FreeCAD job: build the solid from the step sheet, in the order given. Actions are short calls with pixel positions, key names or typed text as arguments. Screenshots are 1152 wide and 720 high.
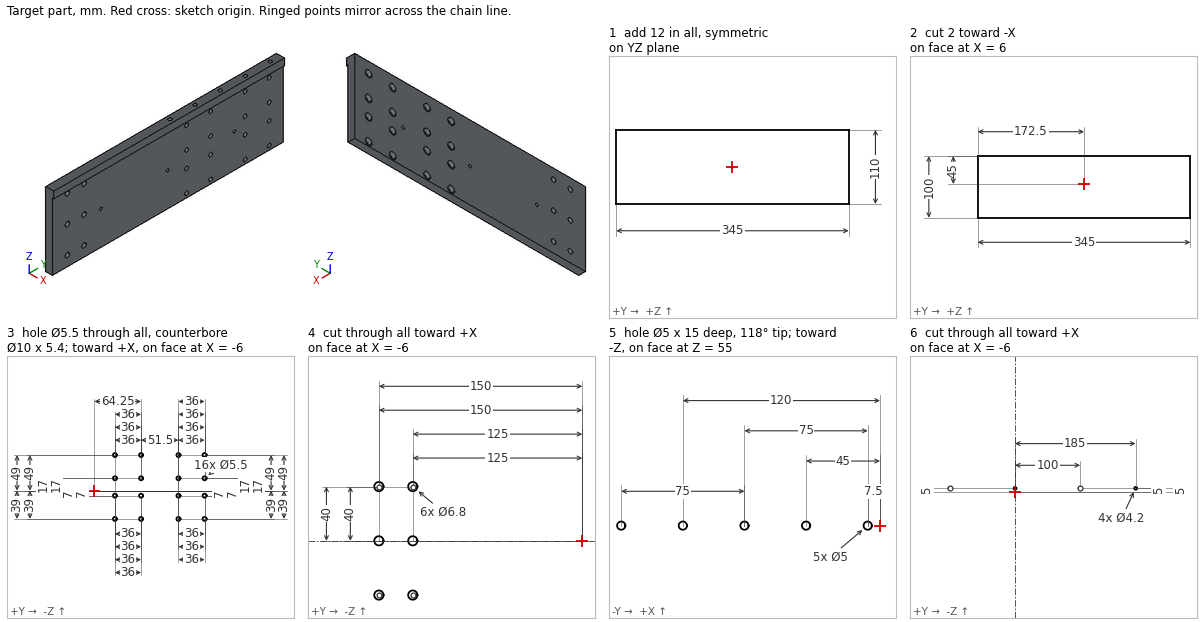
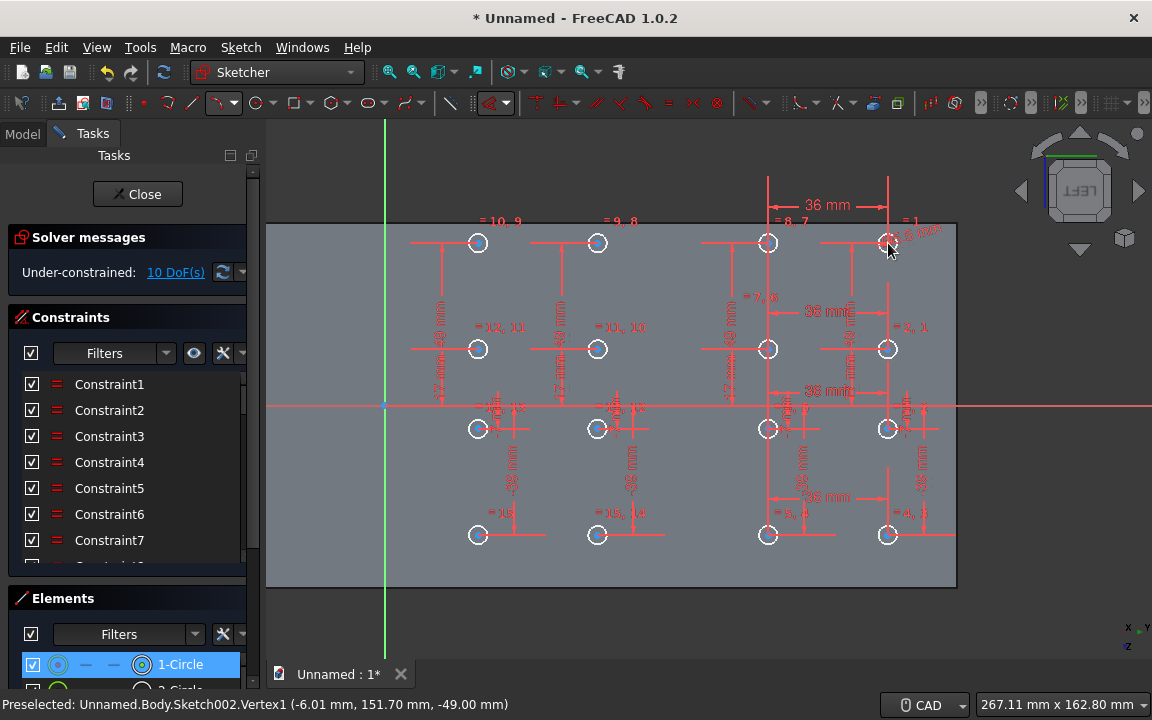
click(768, 243)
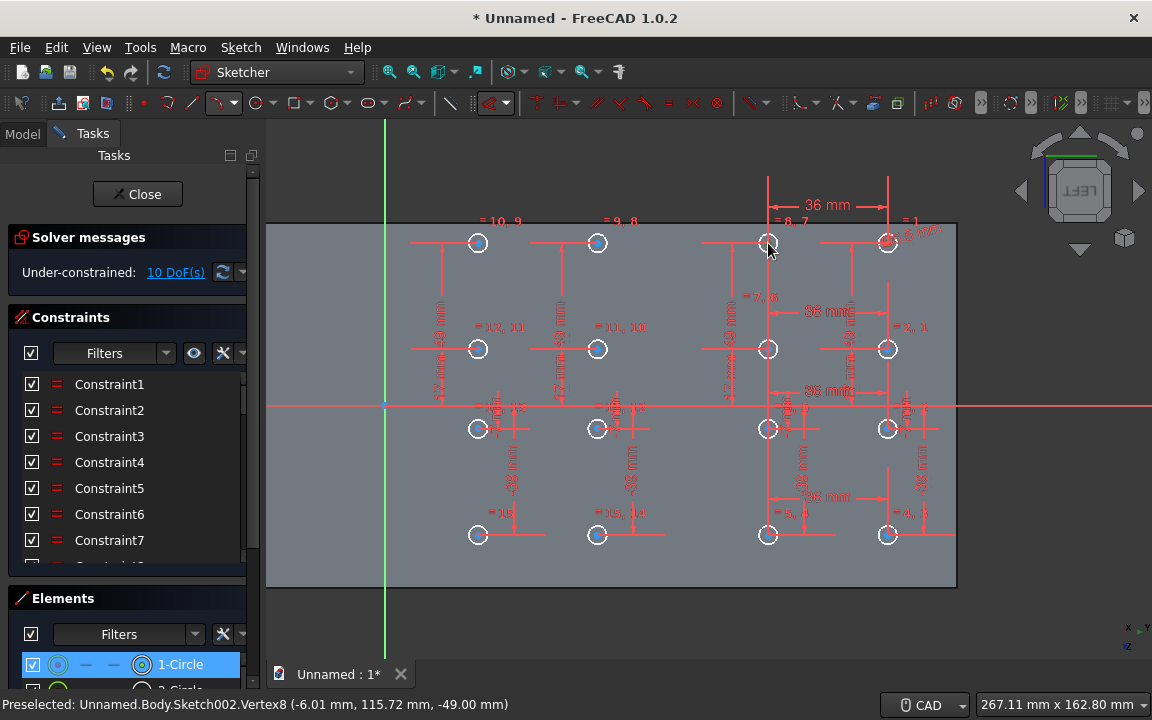
key(l)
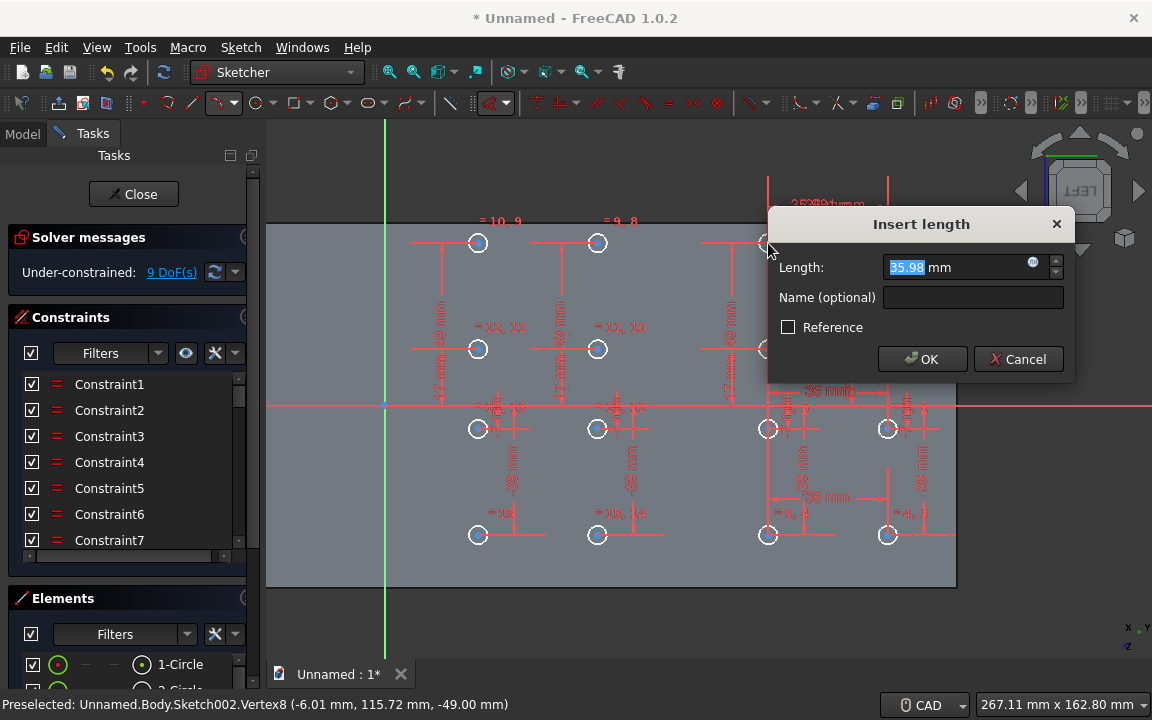
text(36)
key(Return)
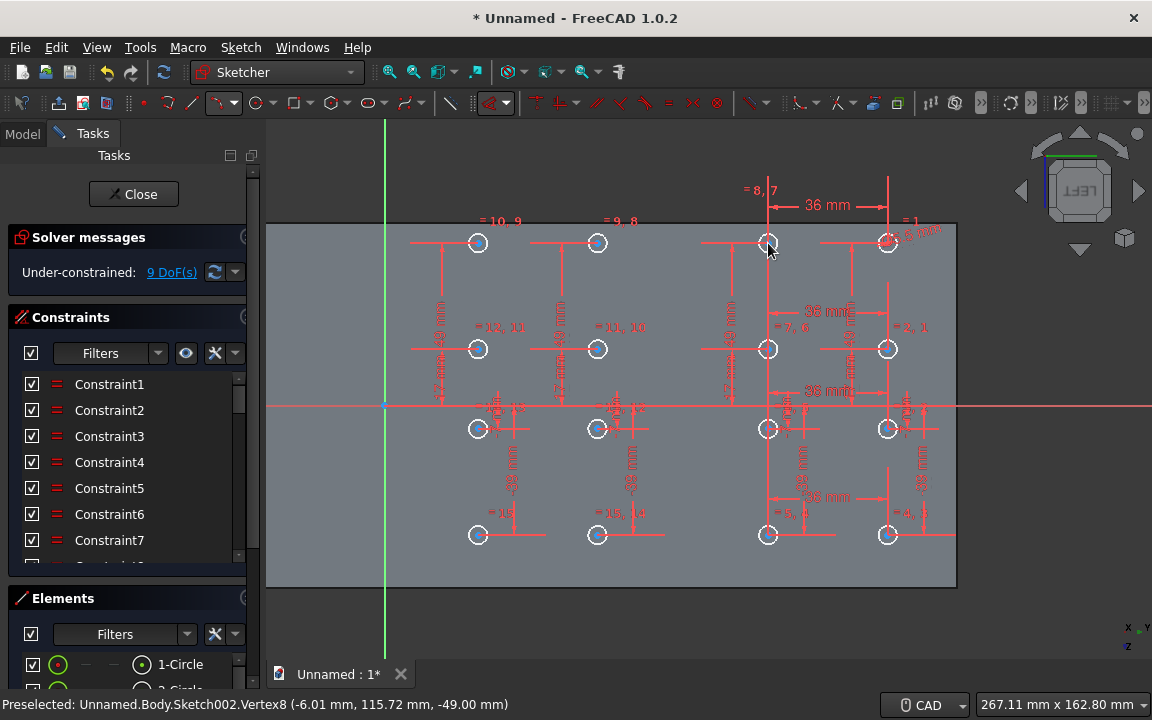
click(598, 243)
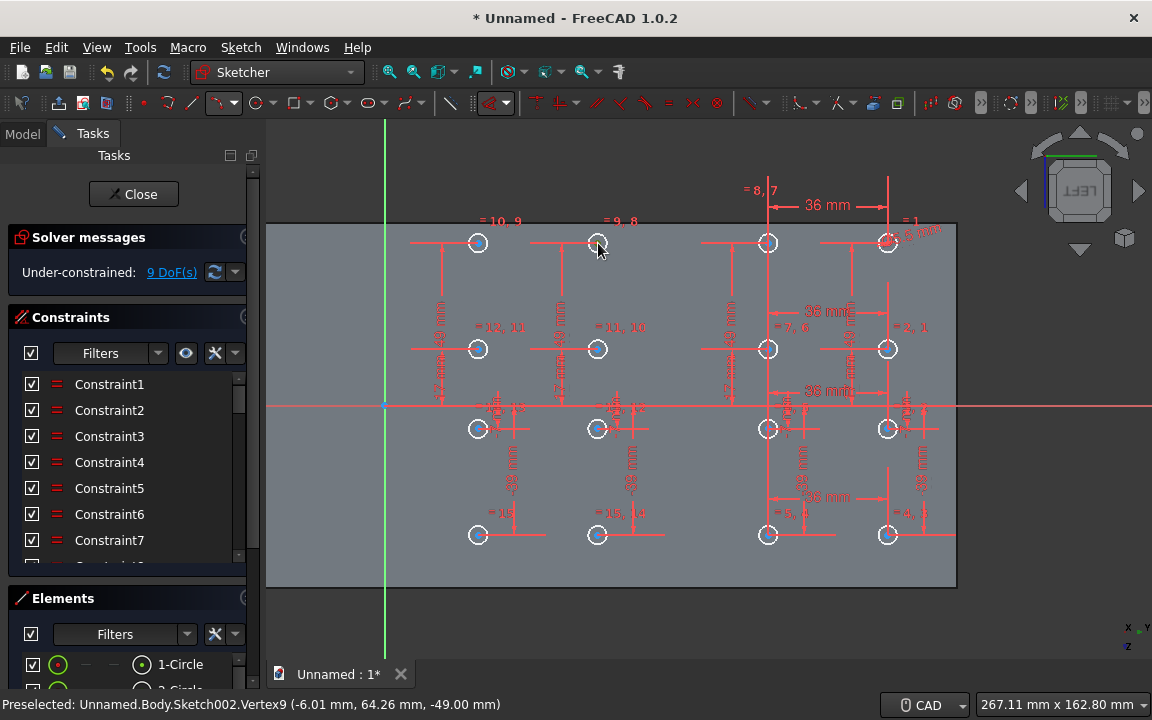
click(478, 243)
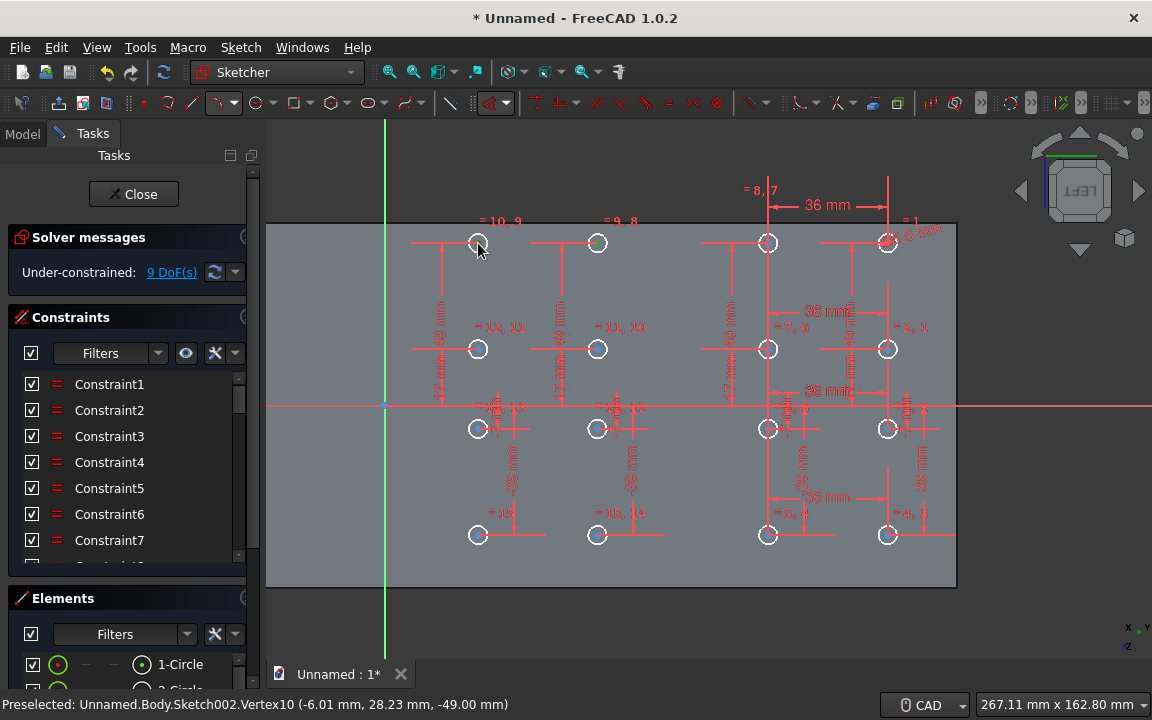
click(508, 104)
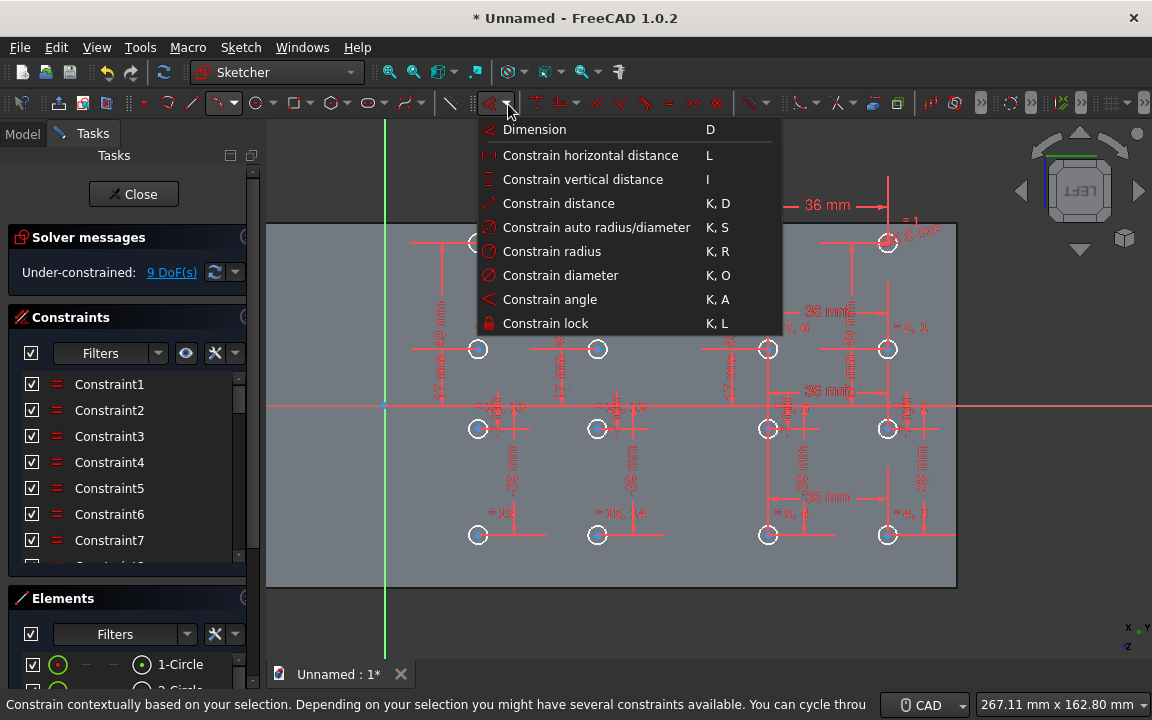
click(630, 155)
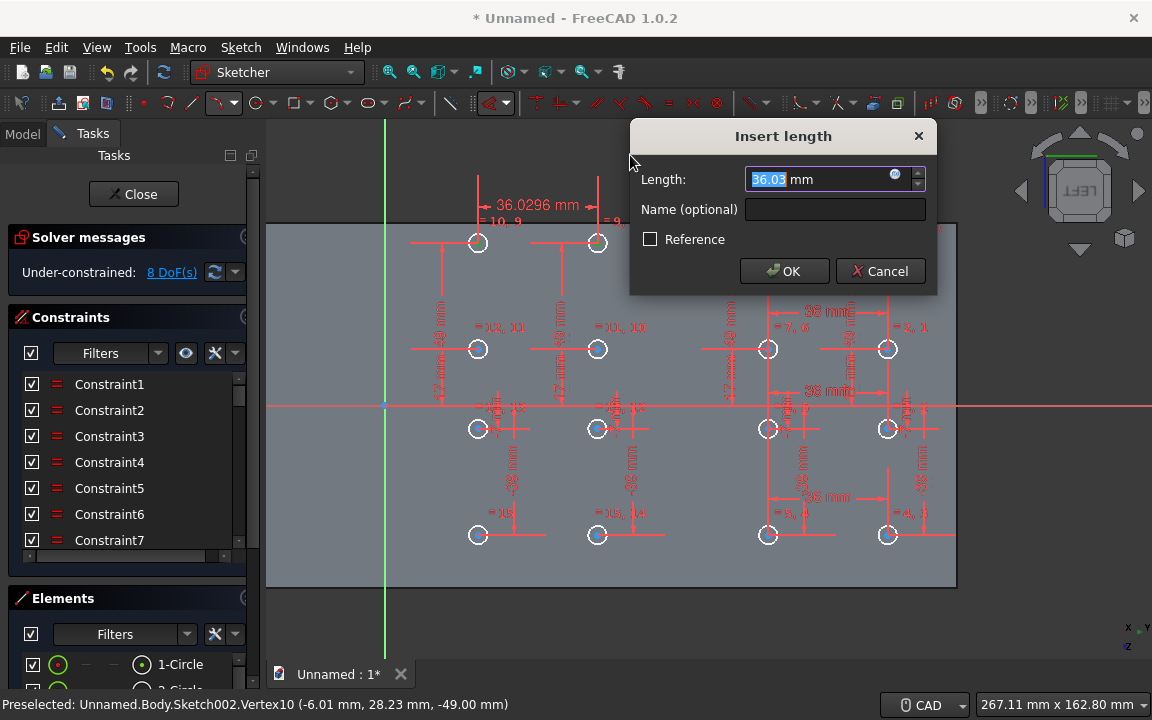
text(36)
key(Return)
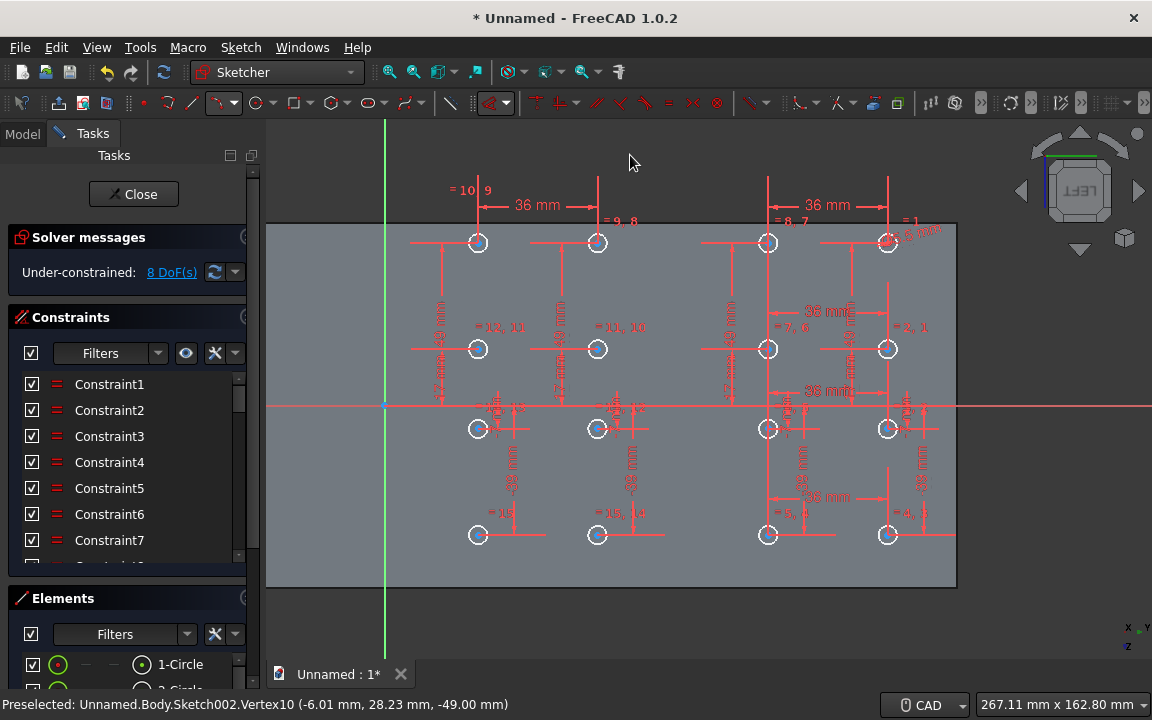
click(478, 243)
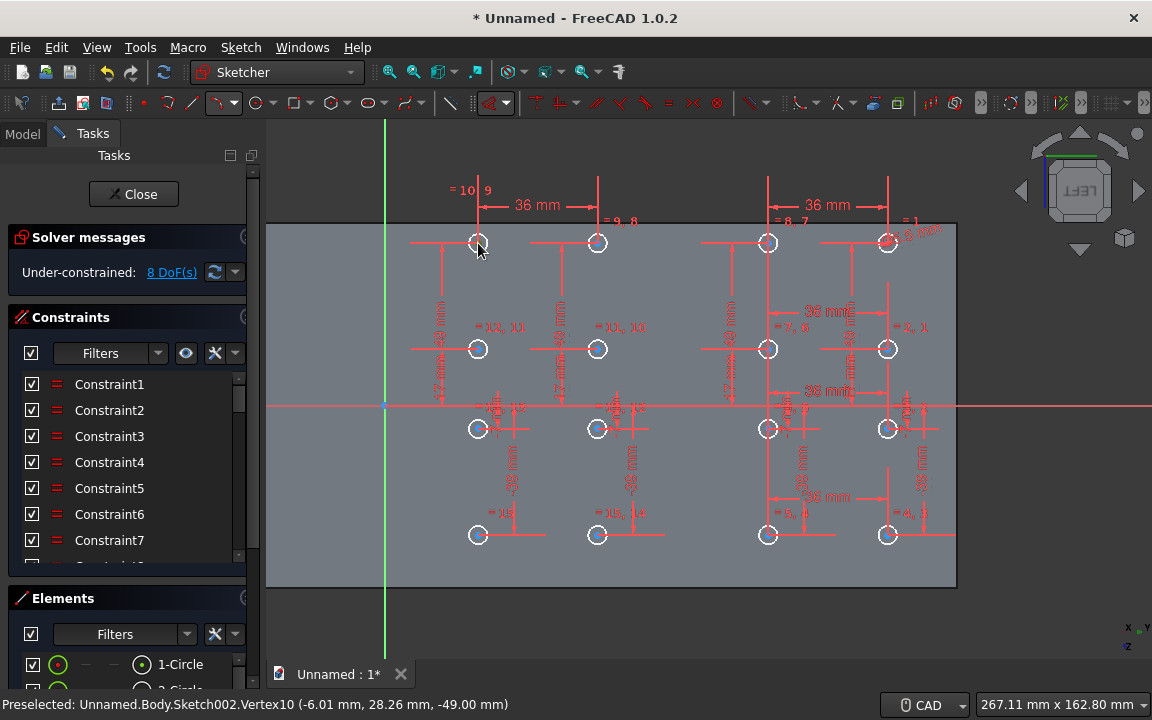
click(598, 349)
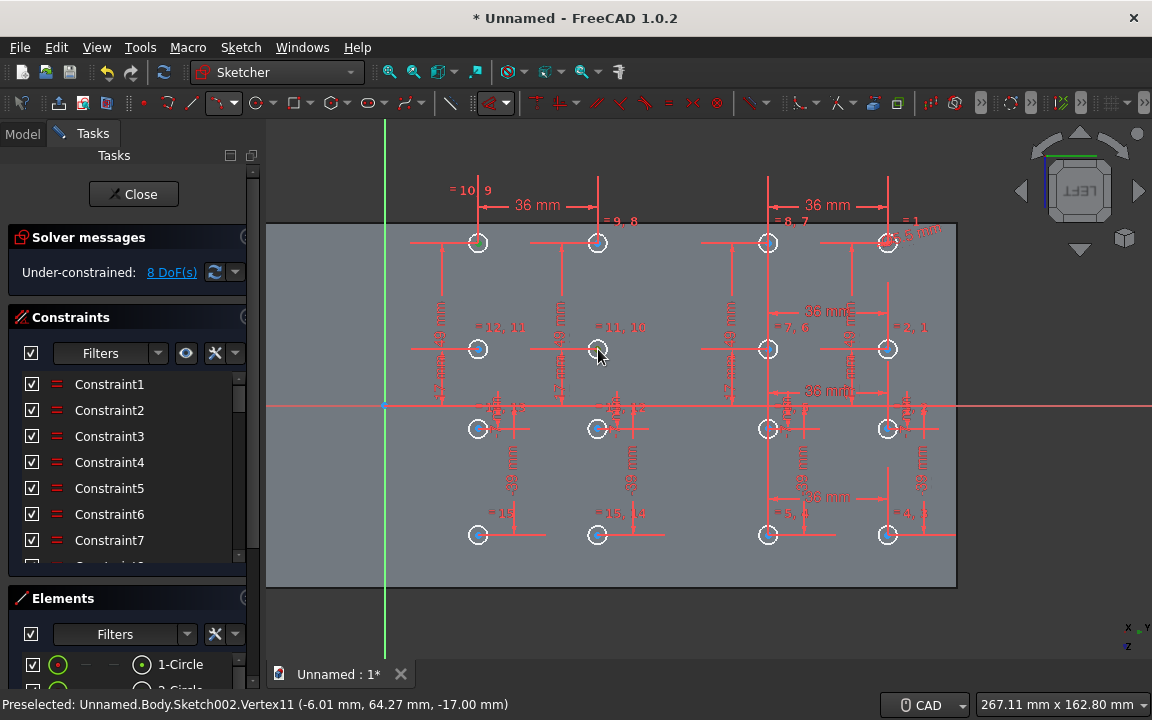
click(508, 104)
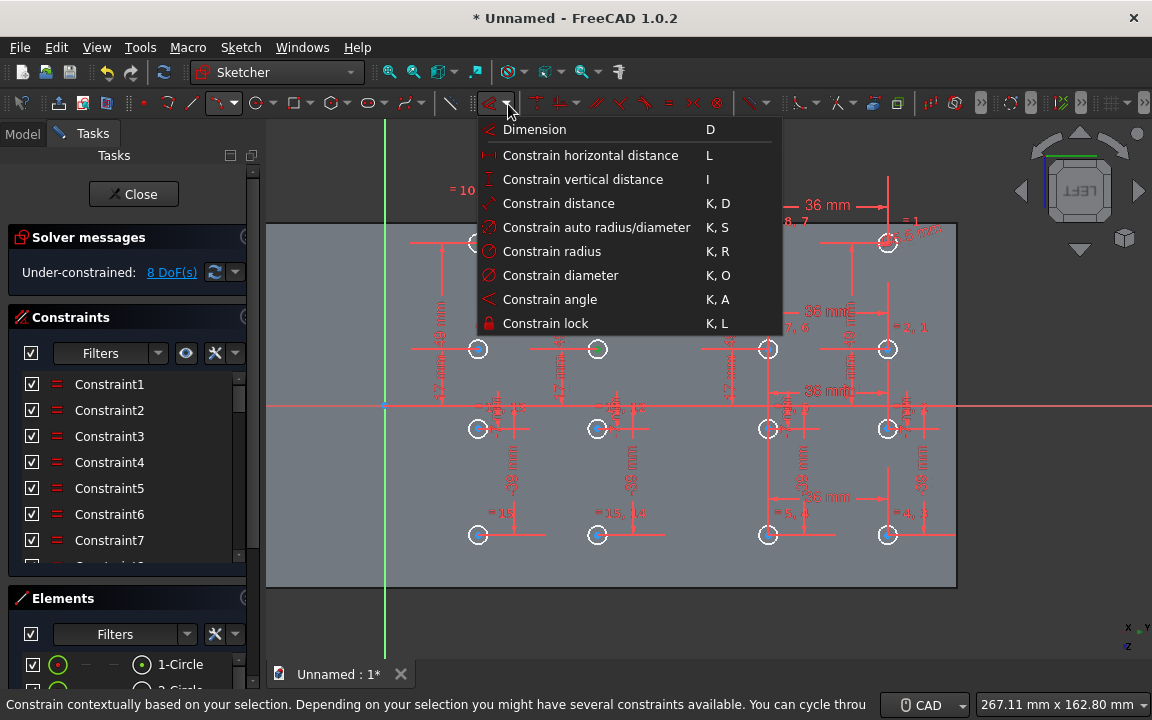
click(630, 155)